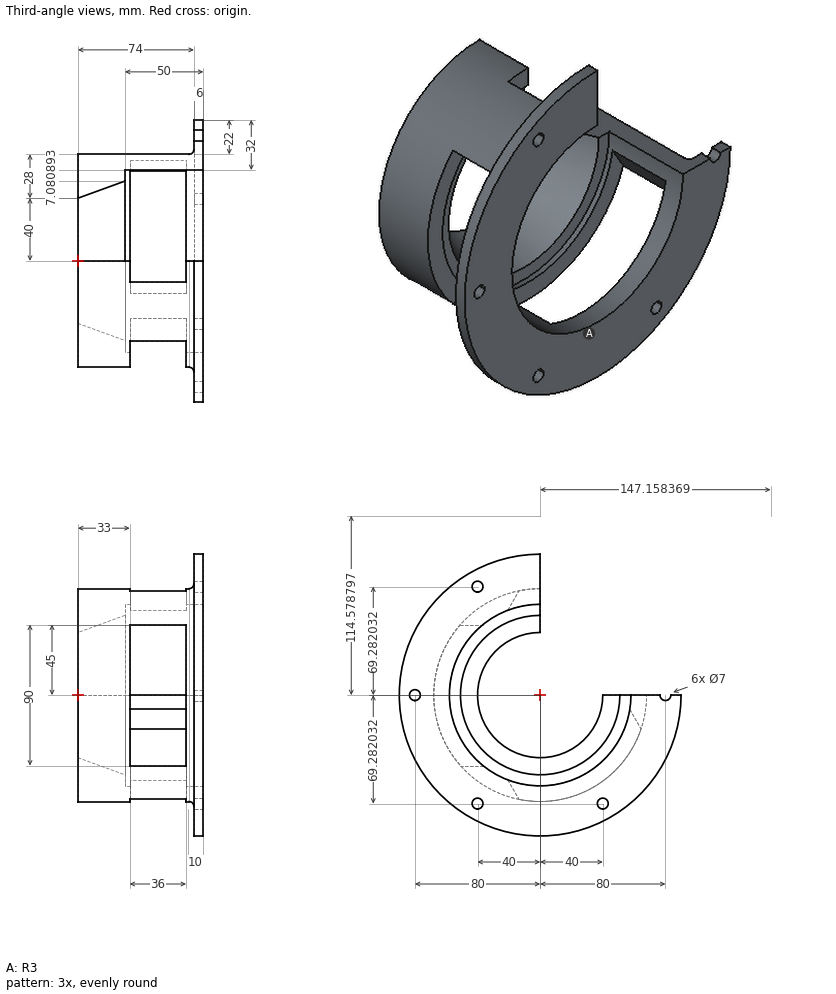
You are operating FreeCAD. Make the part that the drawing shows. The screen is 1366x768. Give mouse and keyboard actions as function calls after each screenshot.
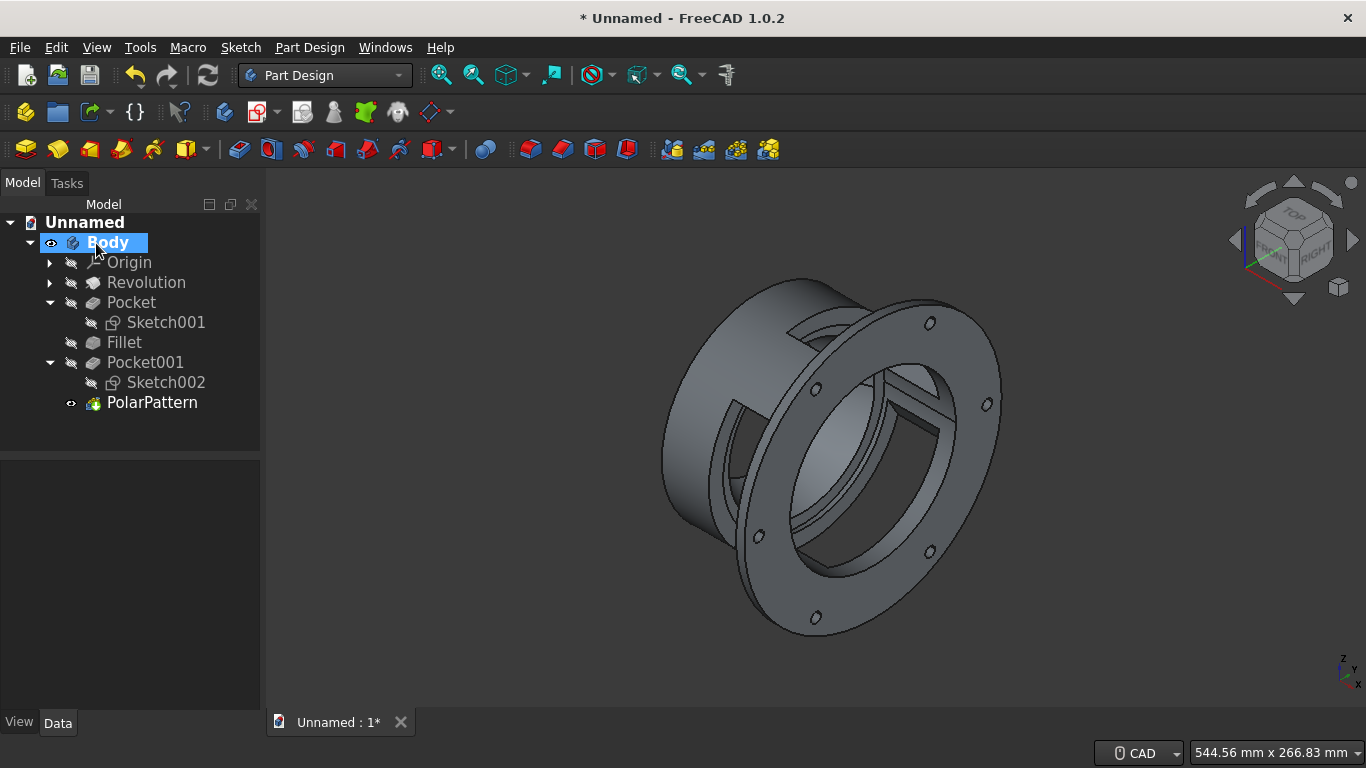
key(6)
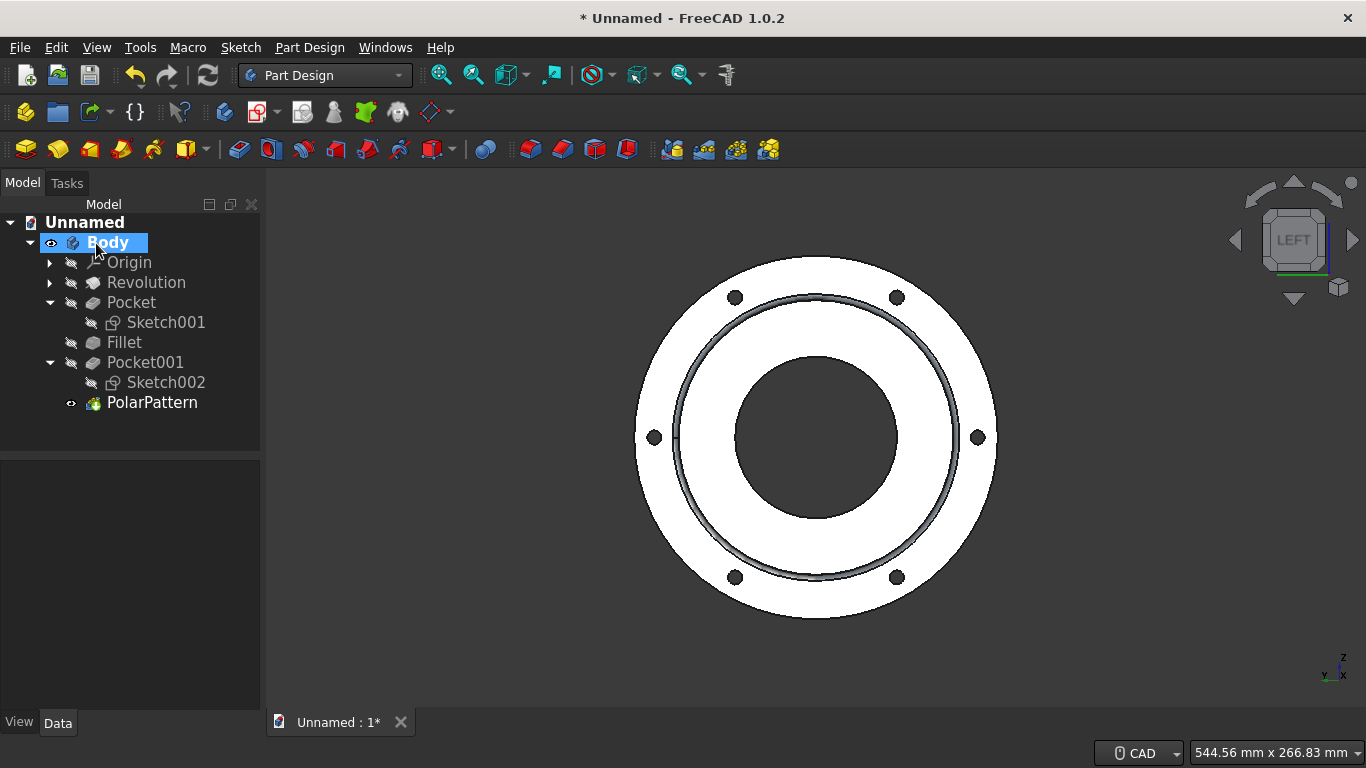
click(894, 515)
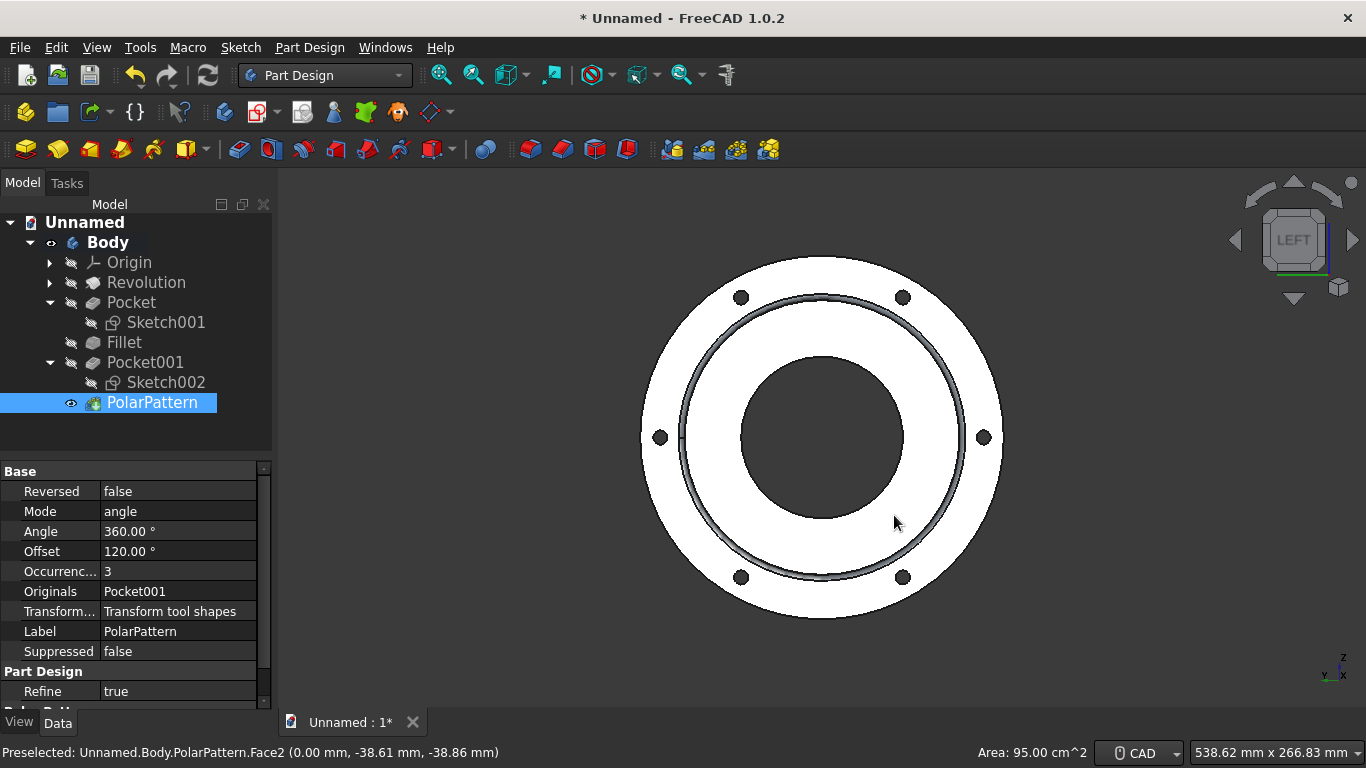
click(258, 112)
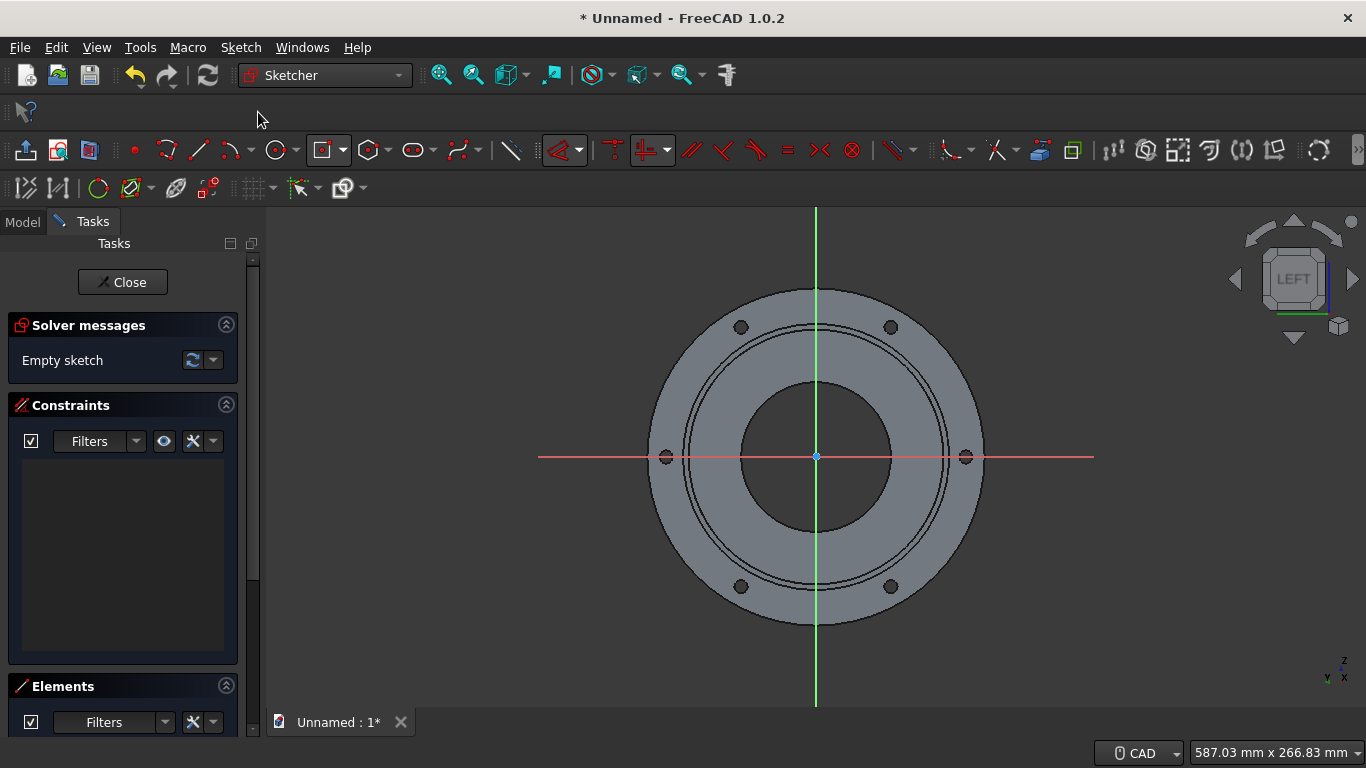
scroll(1061, 679, down, 1)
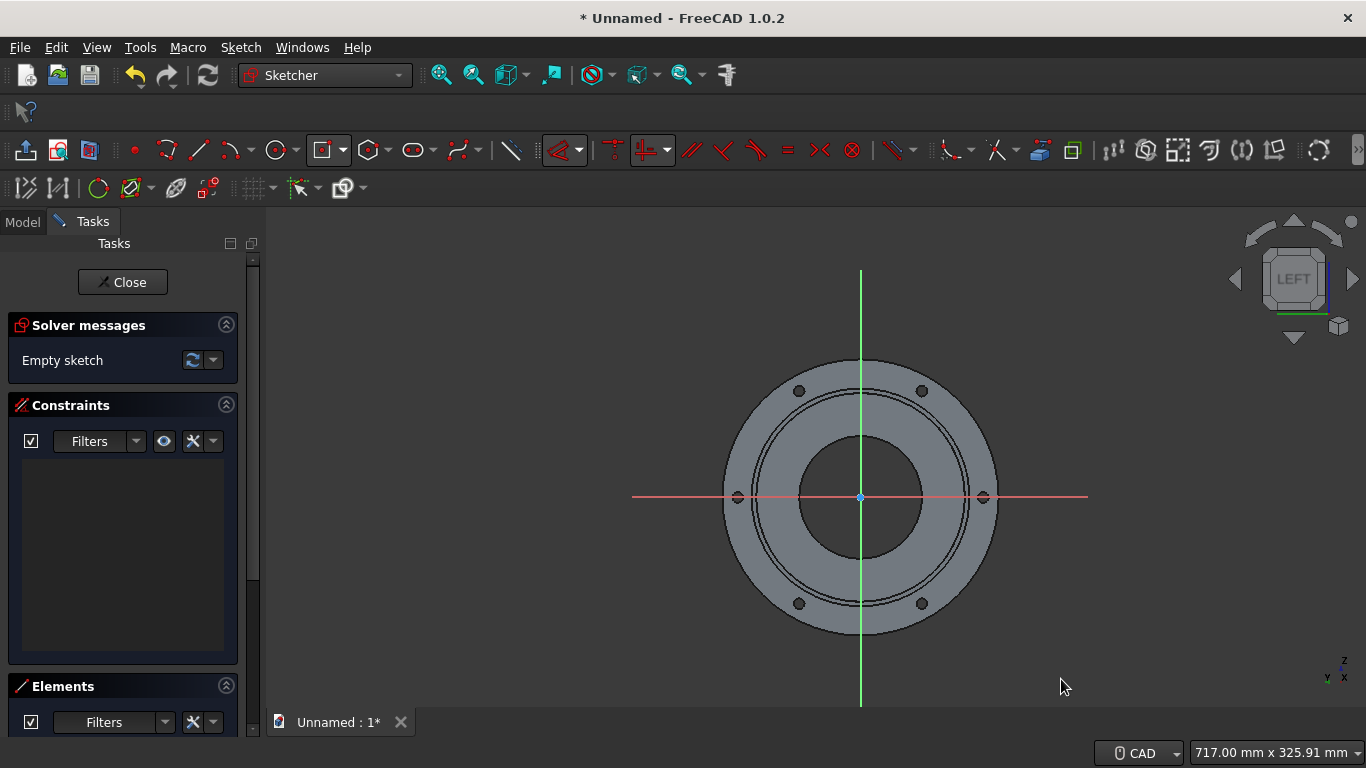
scroll(748, 352, up, 3)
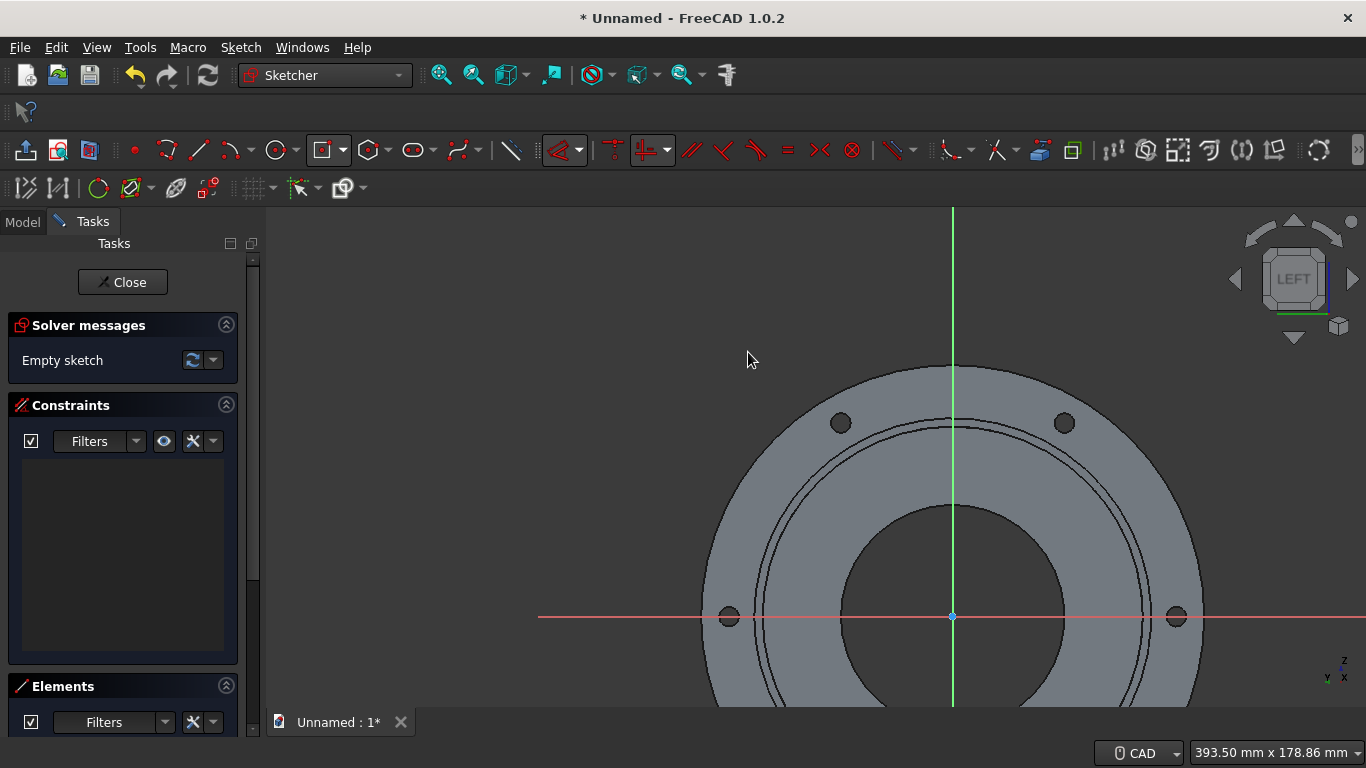
key(g)
key(r)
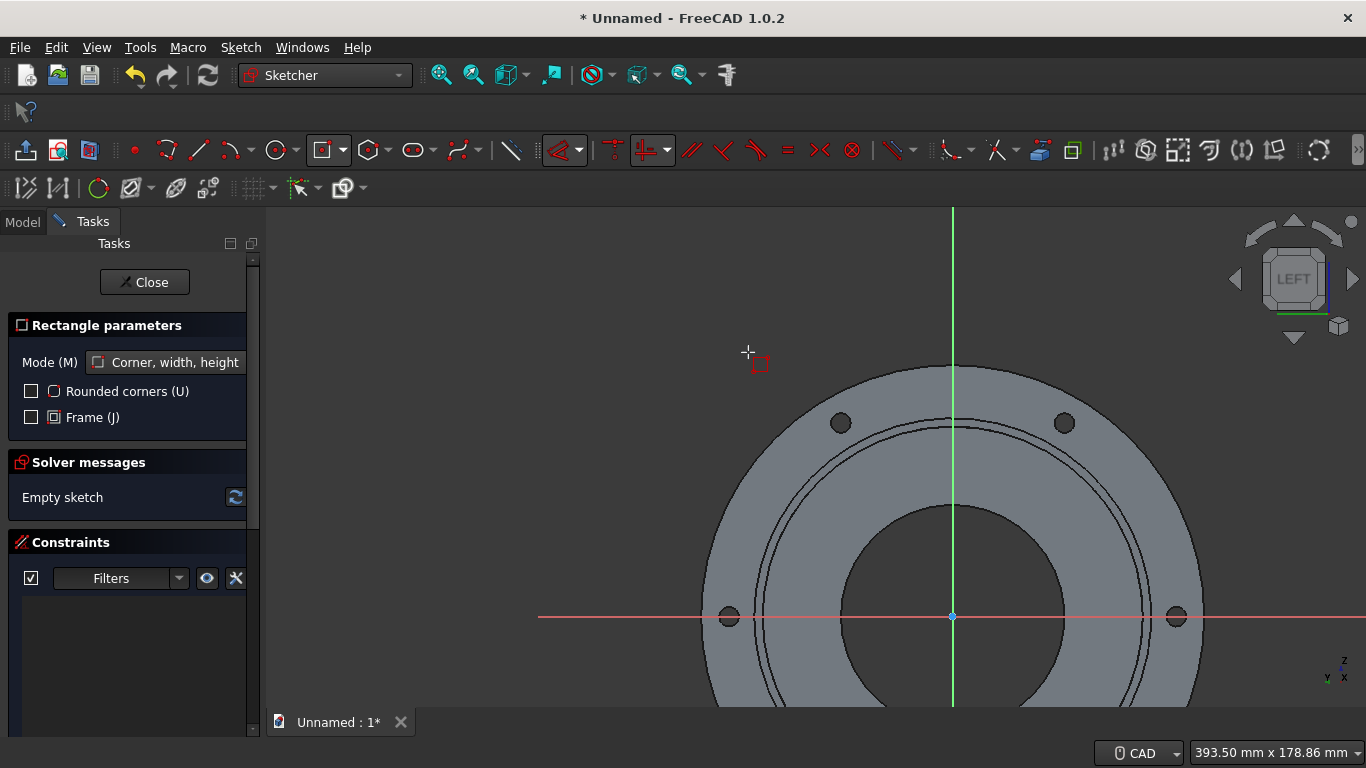
click(953, 617)
click(541, 296)
key(Escape)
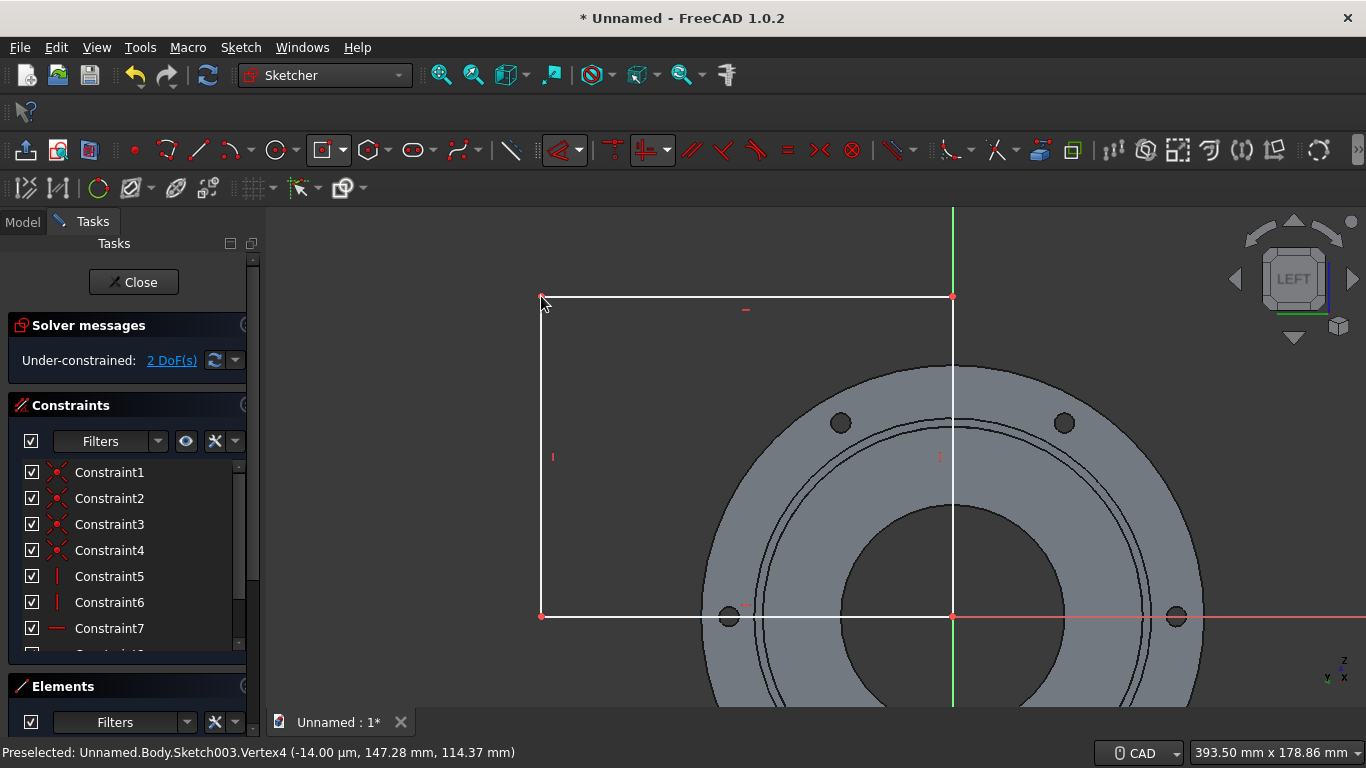
click(953, 521)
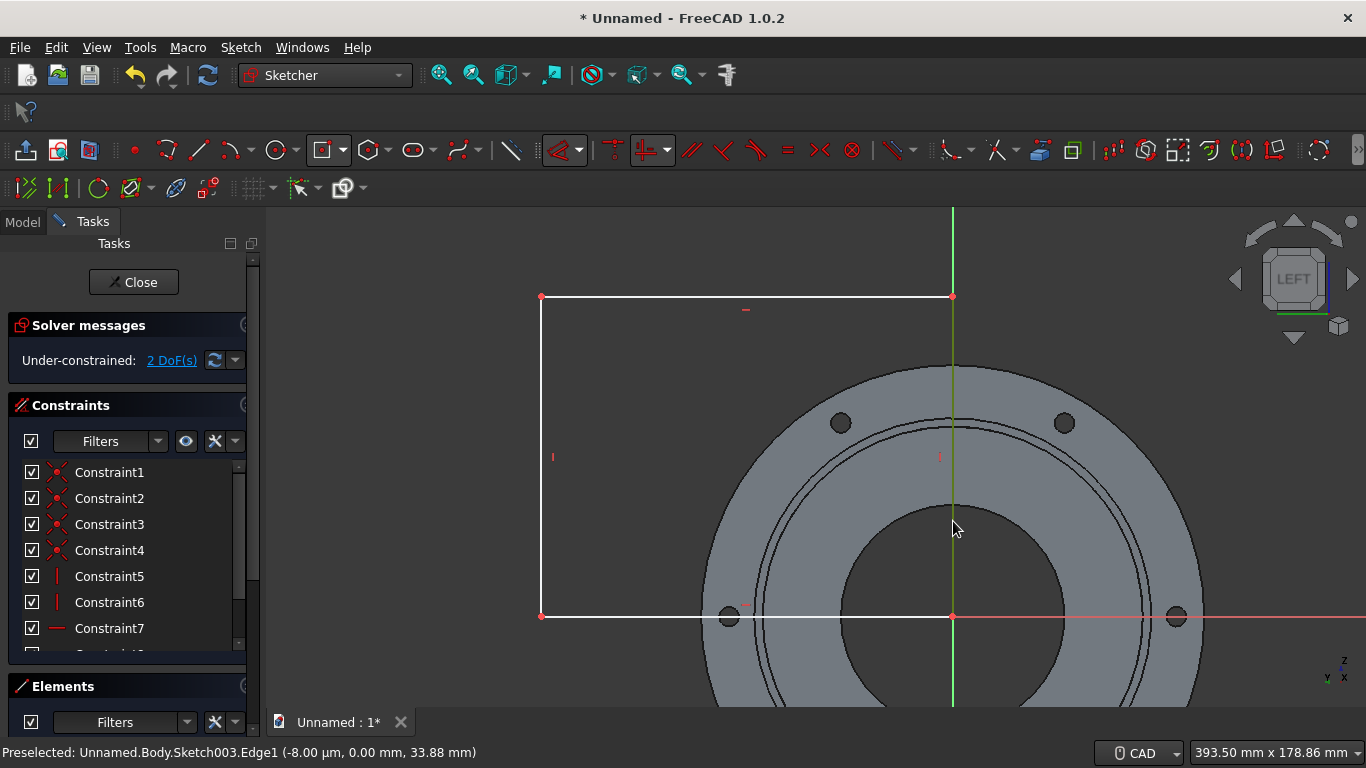
key(i)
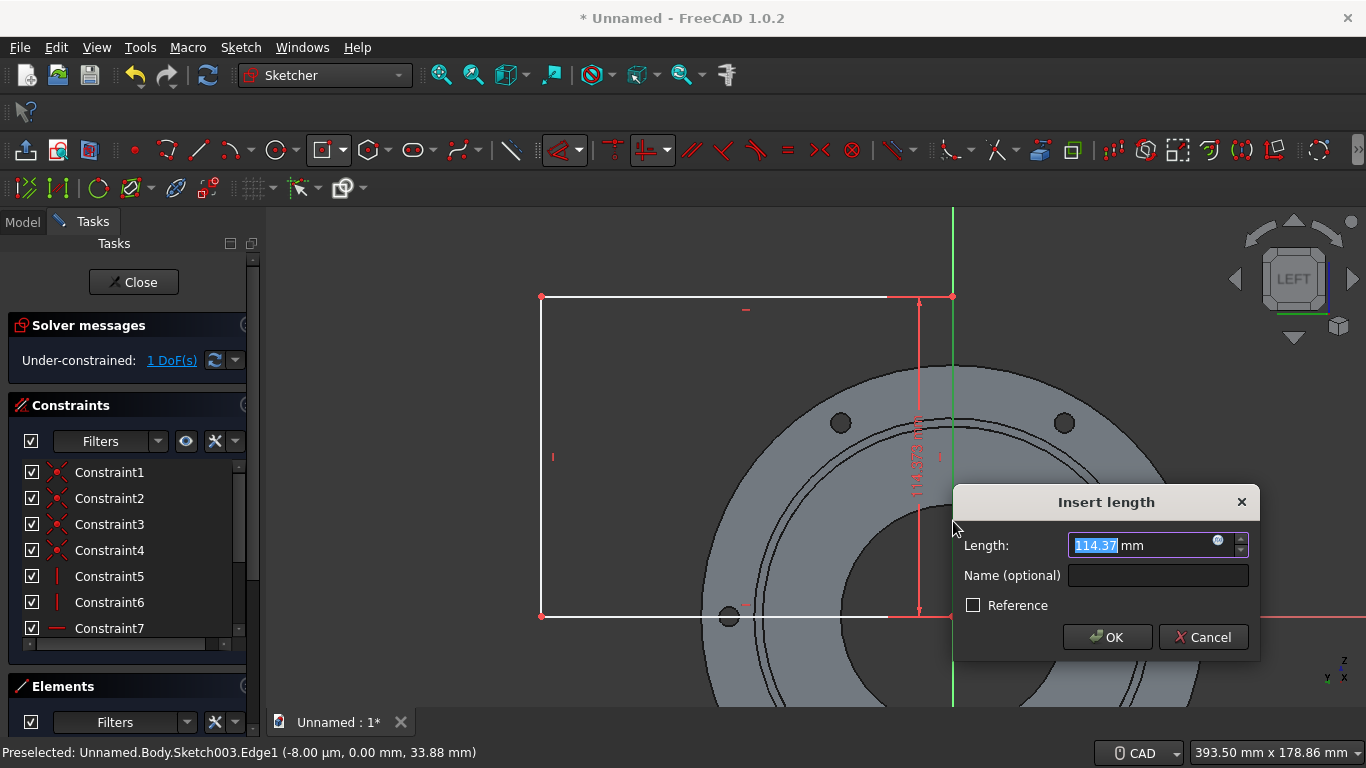
text(114.578797)
key(Return)